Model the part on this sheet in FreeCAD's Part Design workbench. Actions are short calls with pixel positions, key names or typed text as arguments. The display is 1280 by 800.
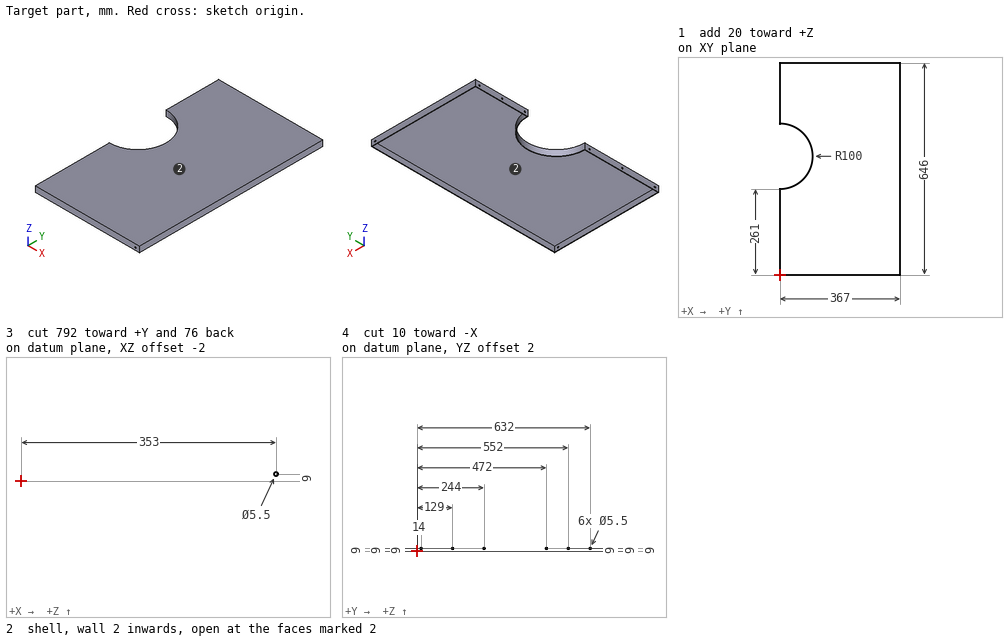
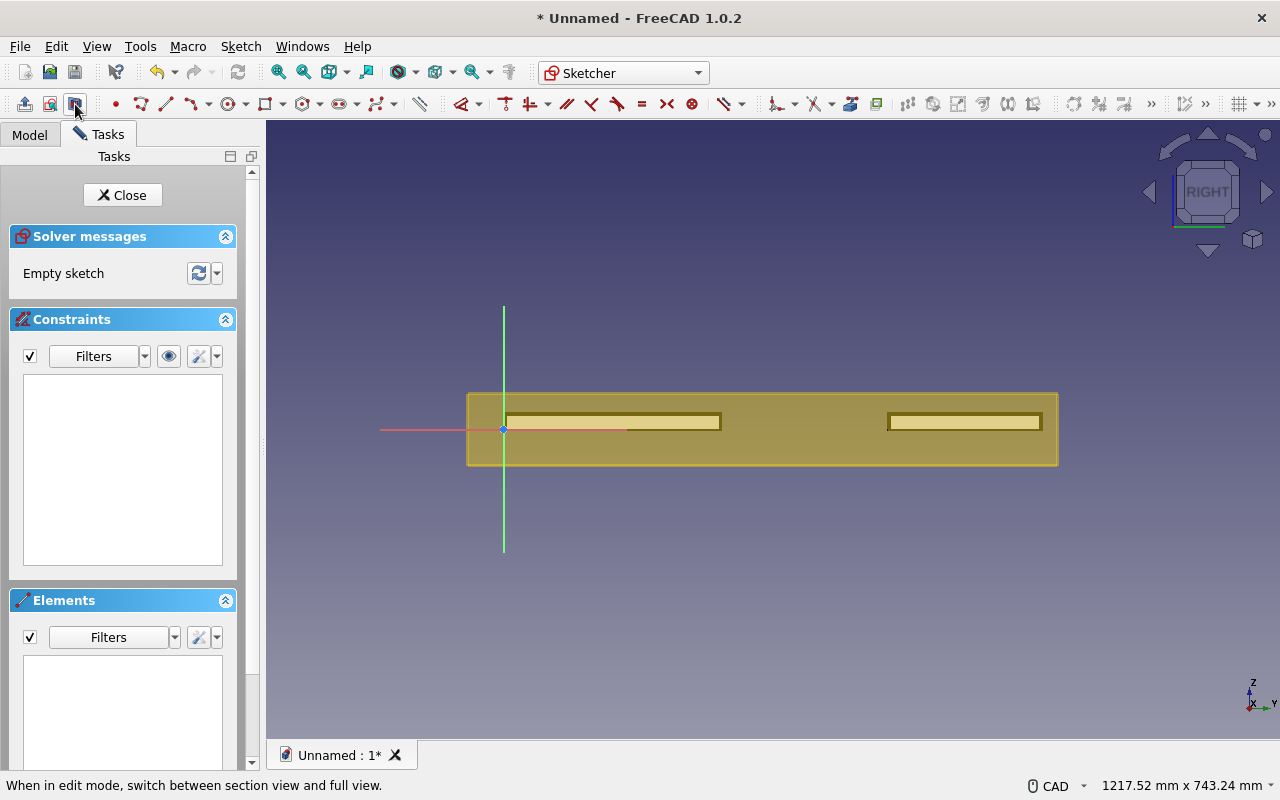
click(228, 104)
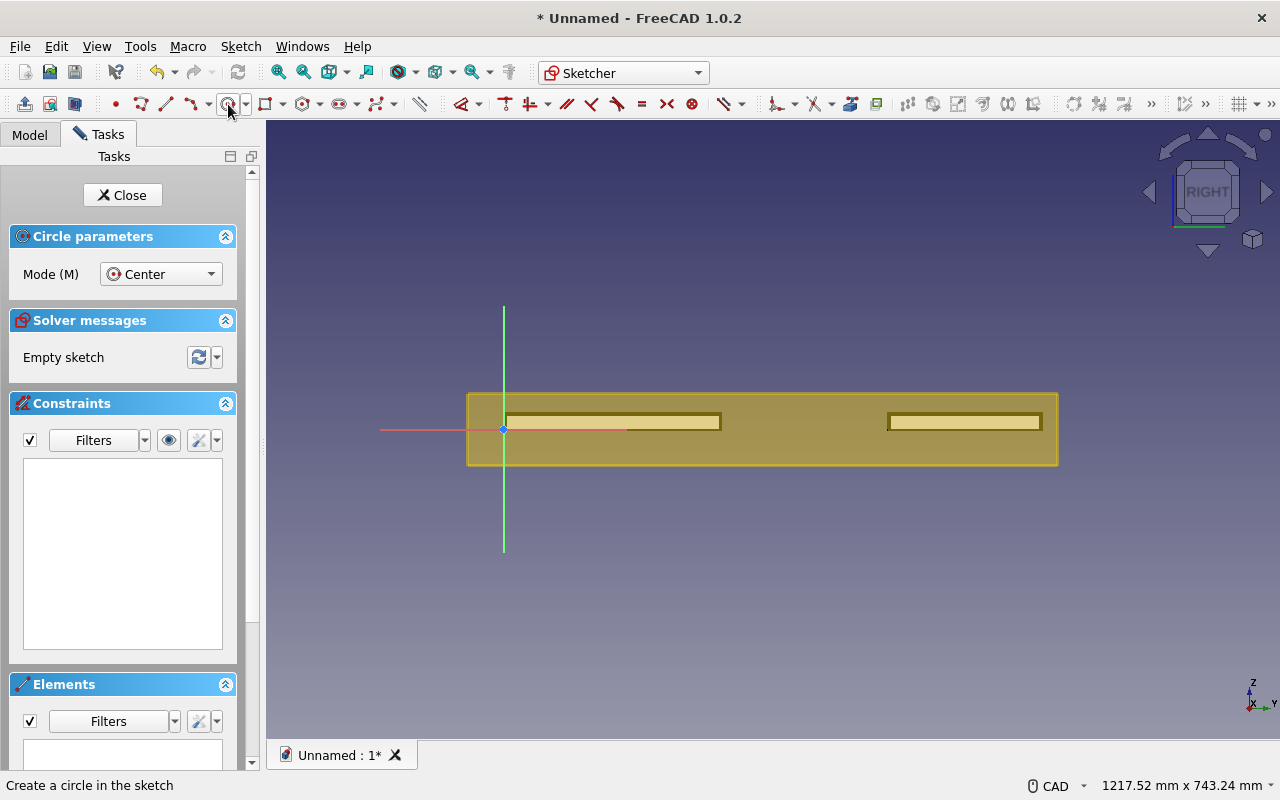
scroll(1030, 422, up, 12)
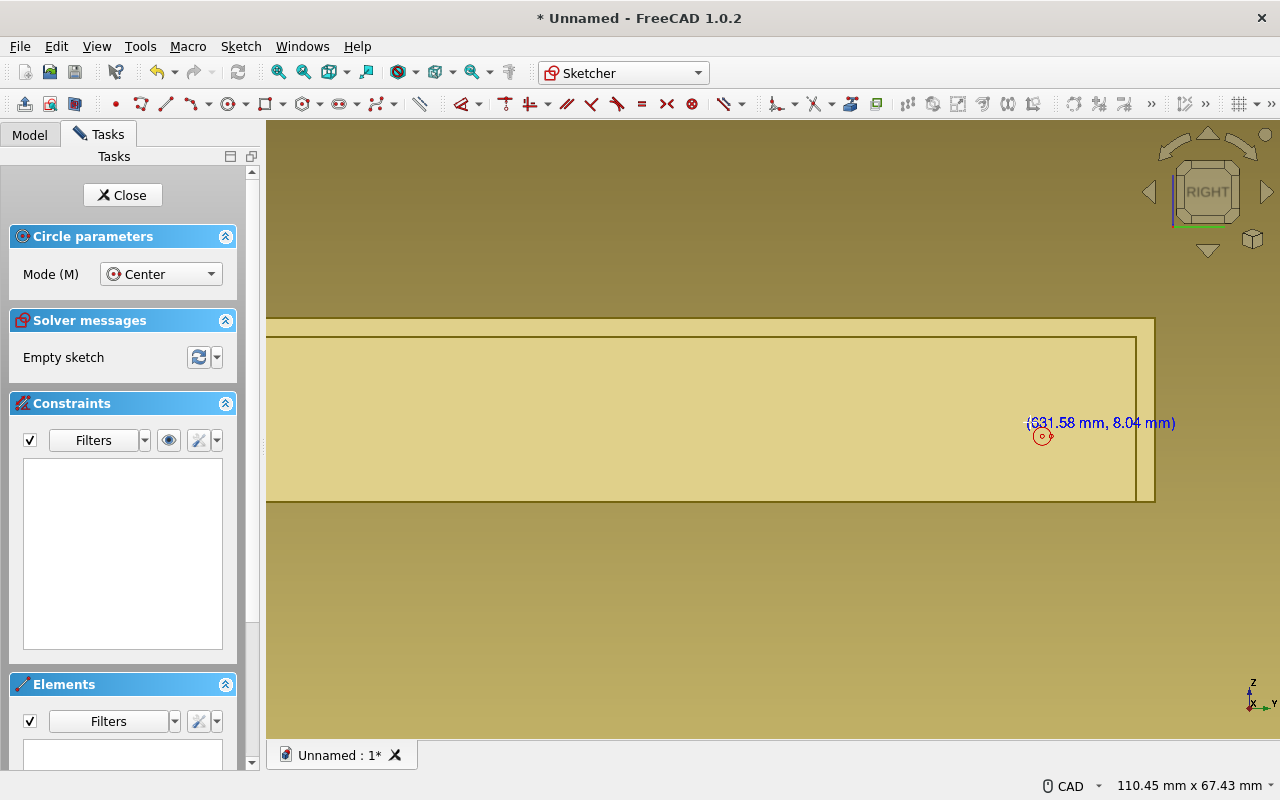
scroll(961, 428, down, 12)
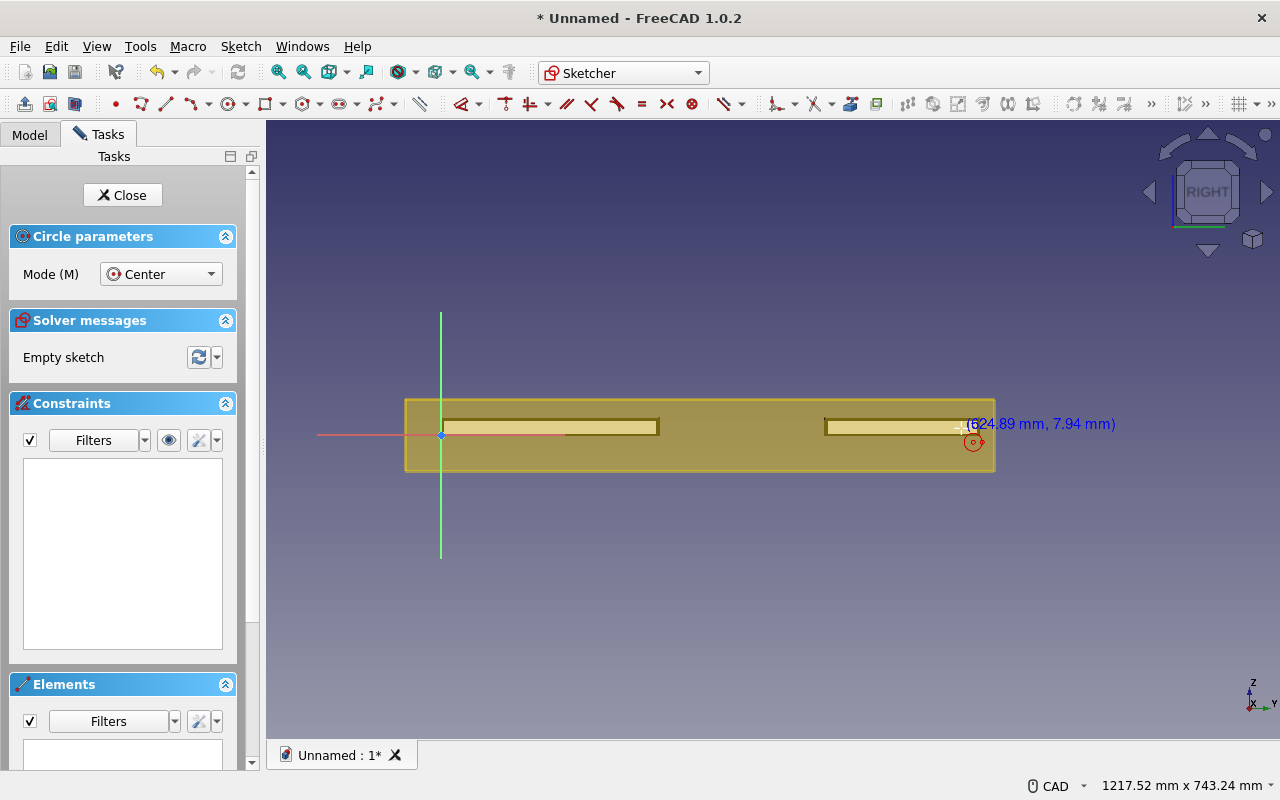
scroll(968, 428, up, 4)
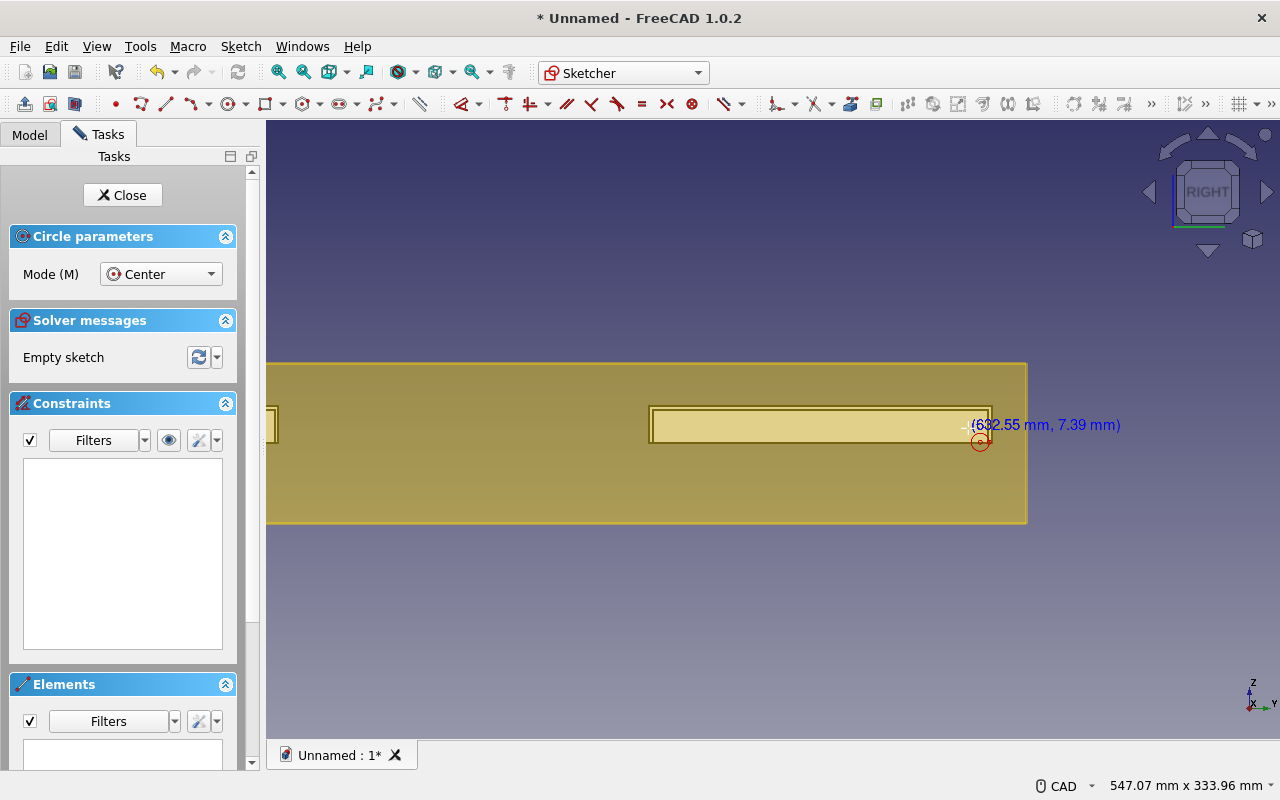
click(966, 427)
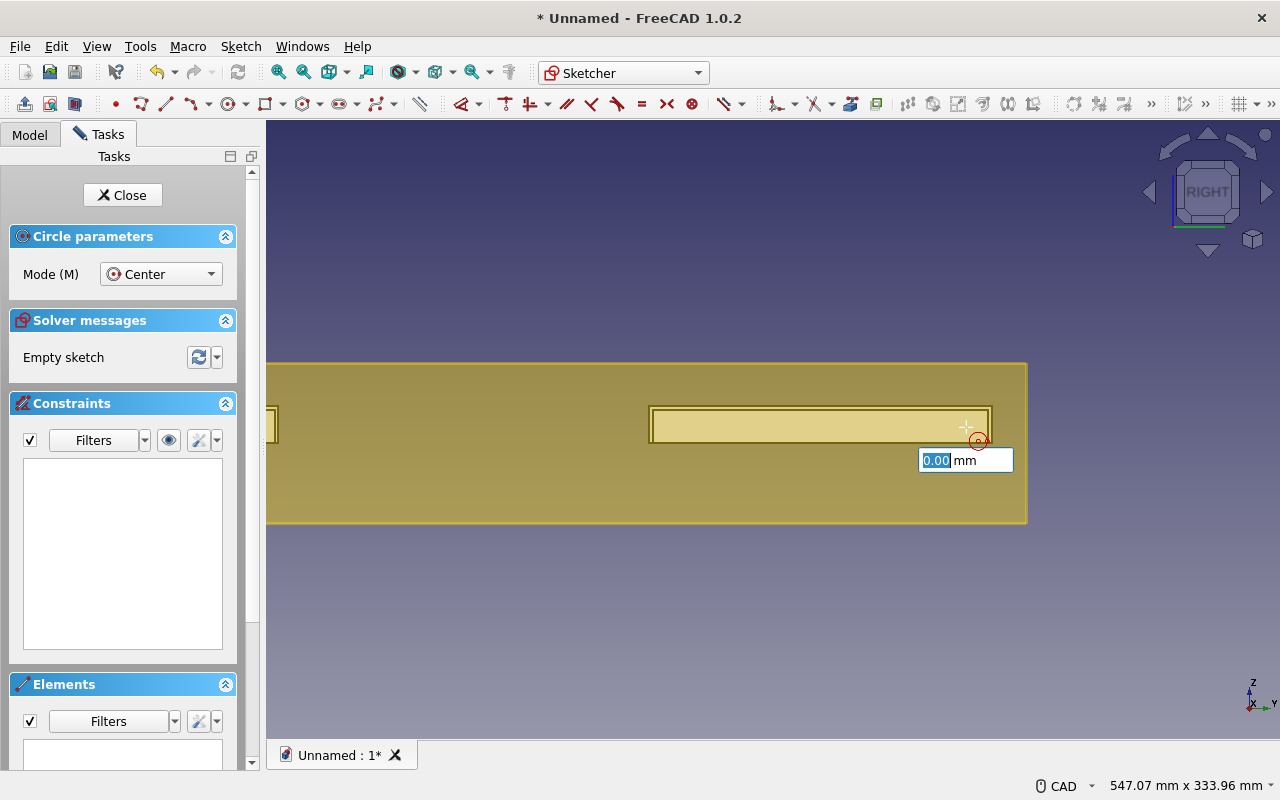
scroll(970, 423, up, 6)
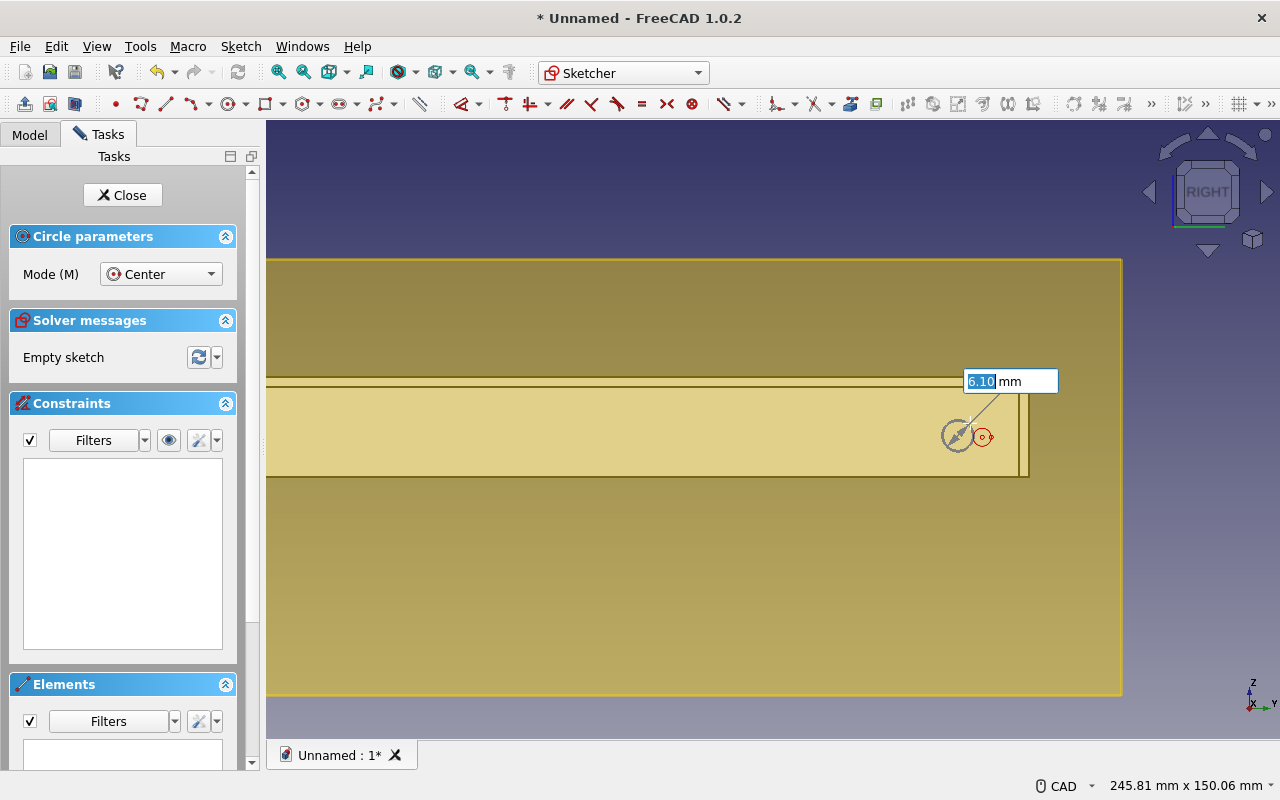
click(968, 422)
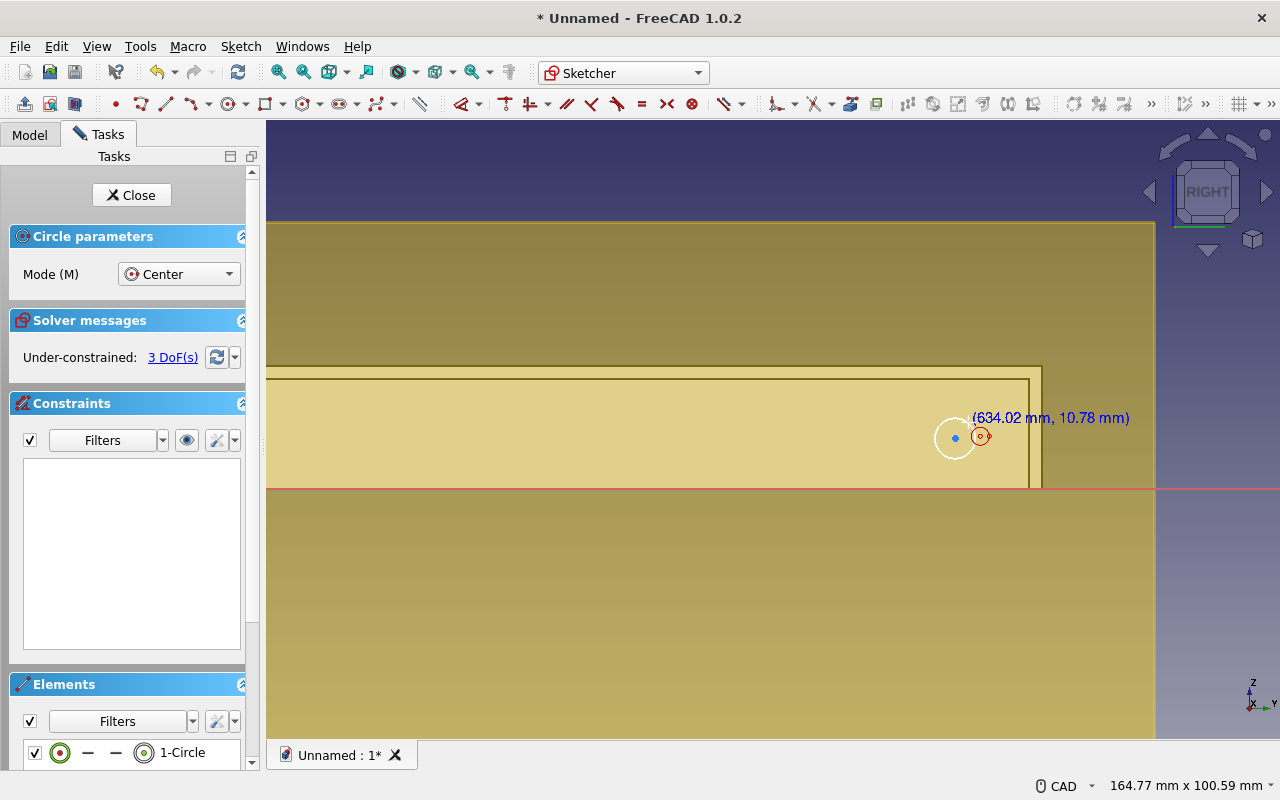
scroll(463, 434, up, 2)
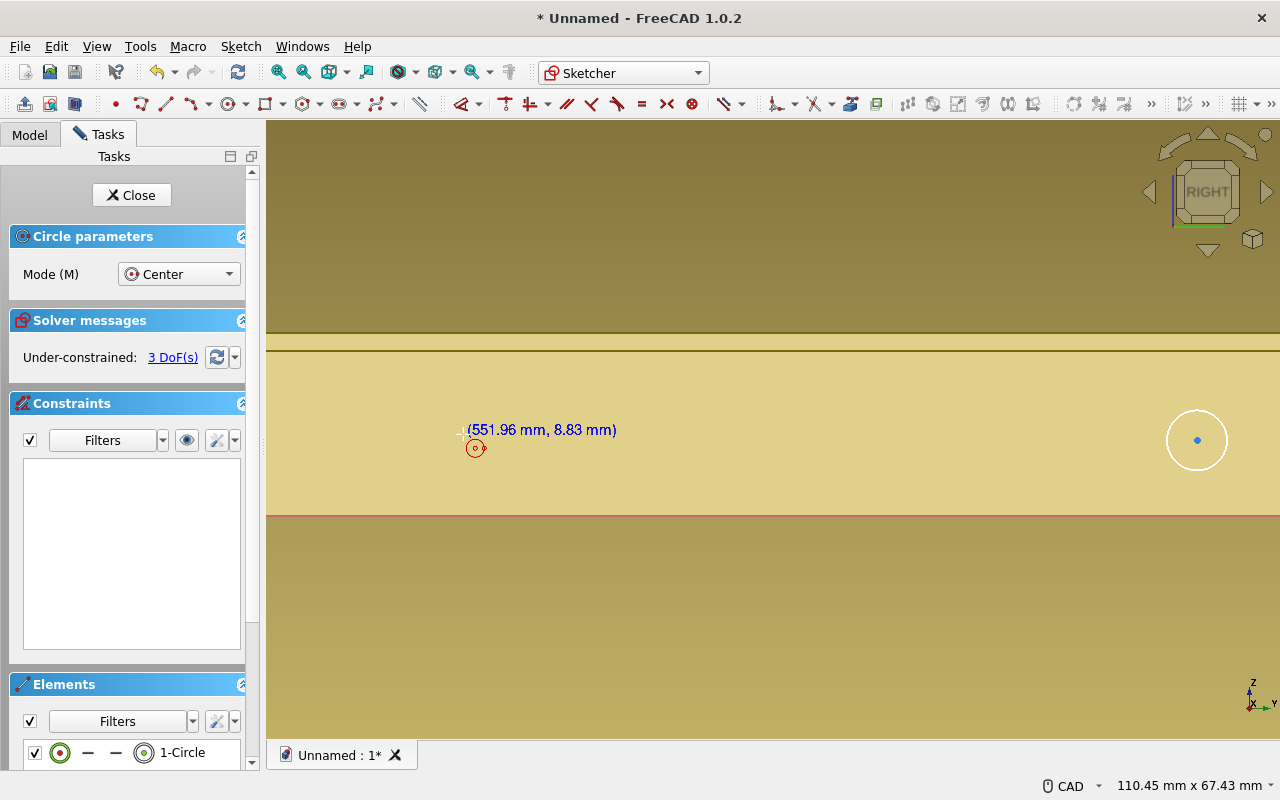
scroll(943, 426, down, 12)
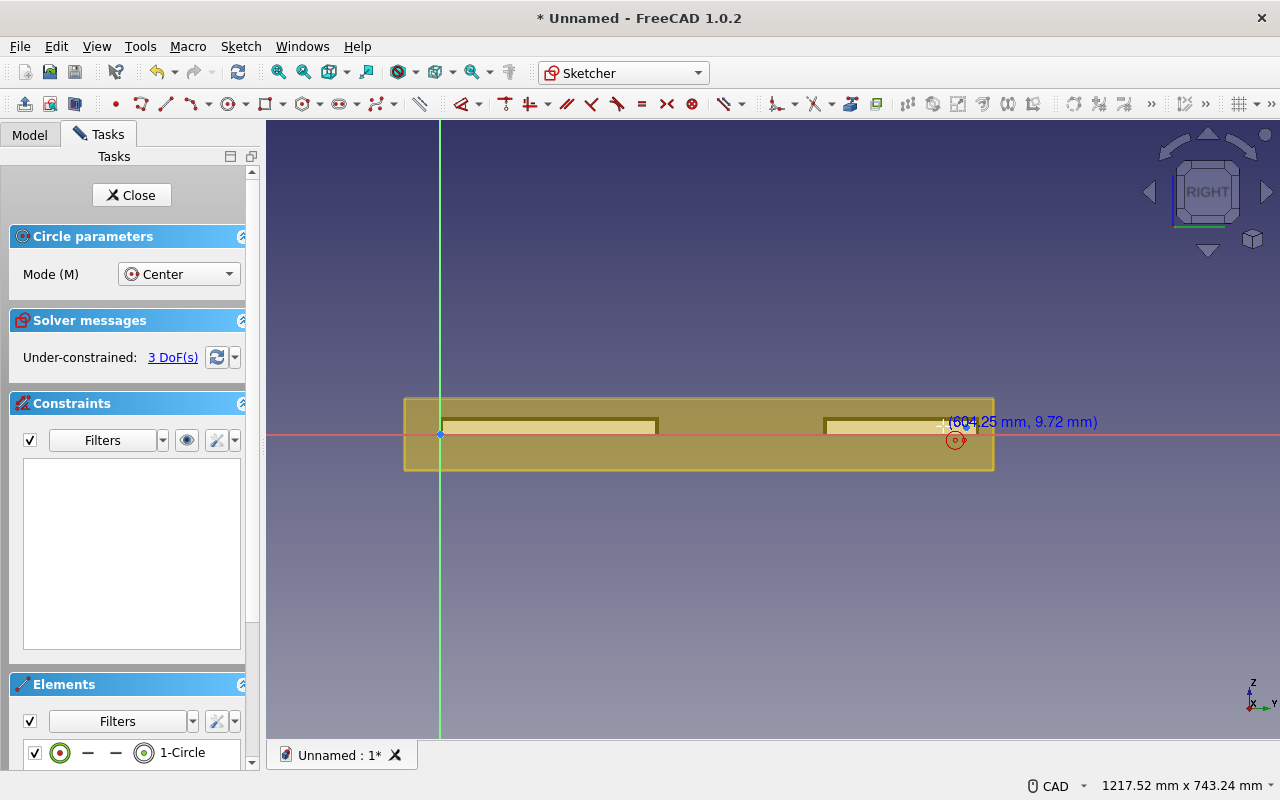
scroll(900, 427, up, 4)